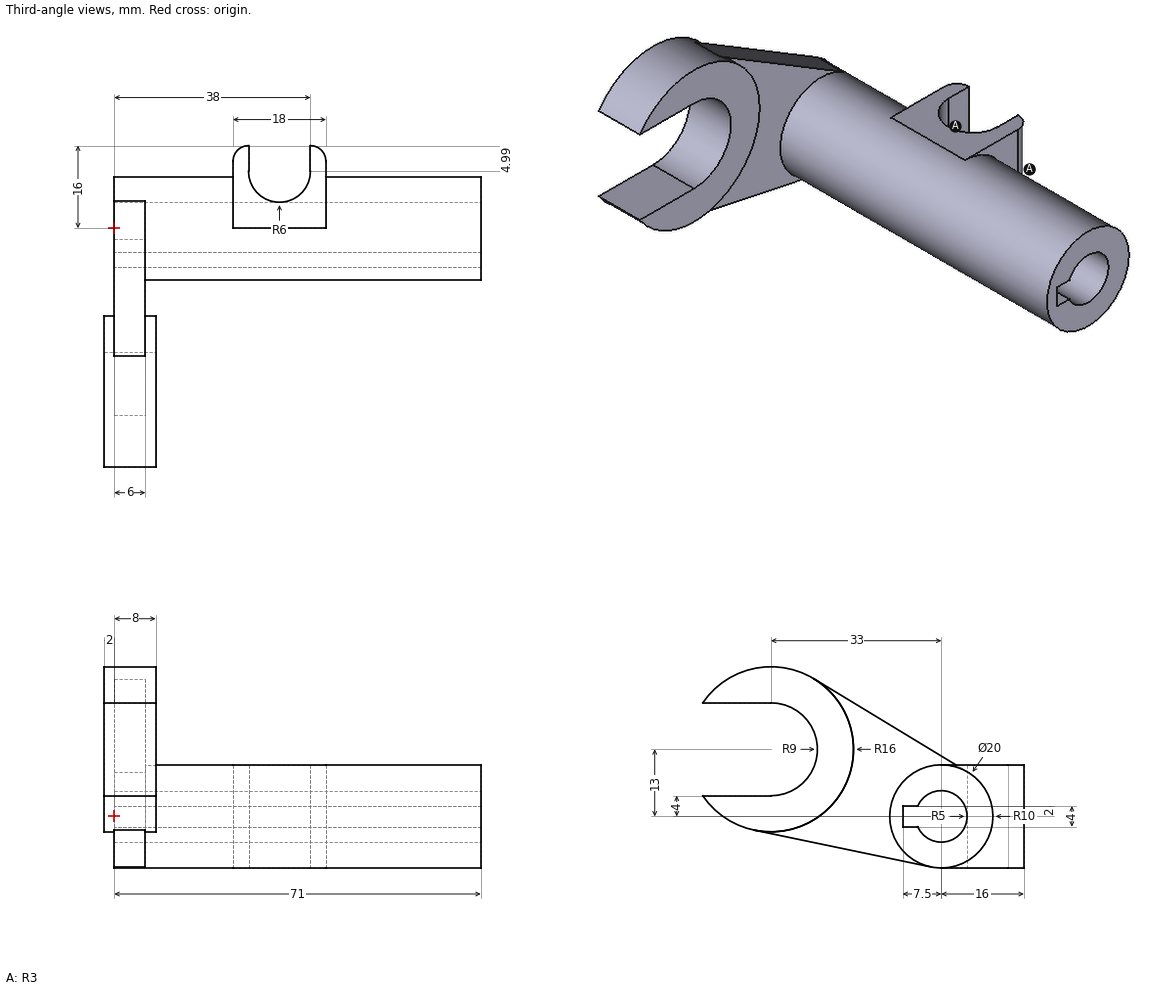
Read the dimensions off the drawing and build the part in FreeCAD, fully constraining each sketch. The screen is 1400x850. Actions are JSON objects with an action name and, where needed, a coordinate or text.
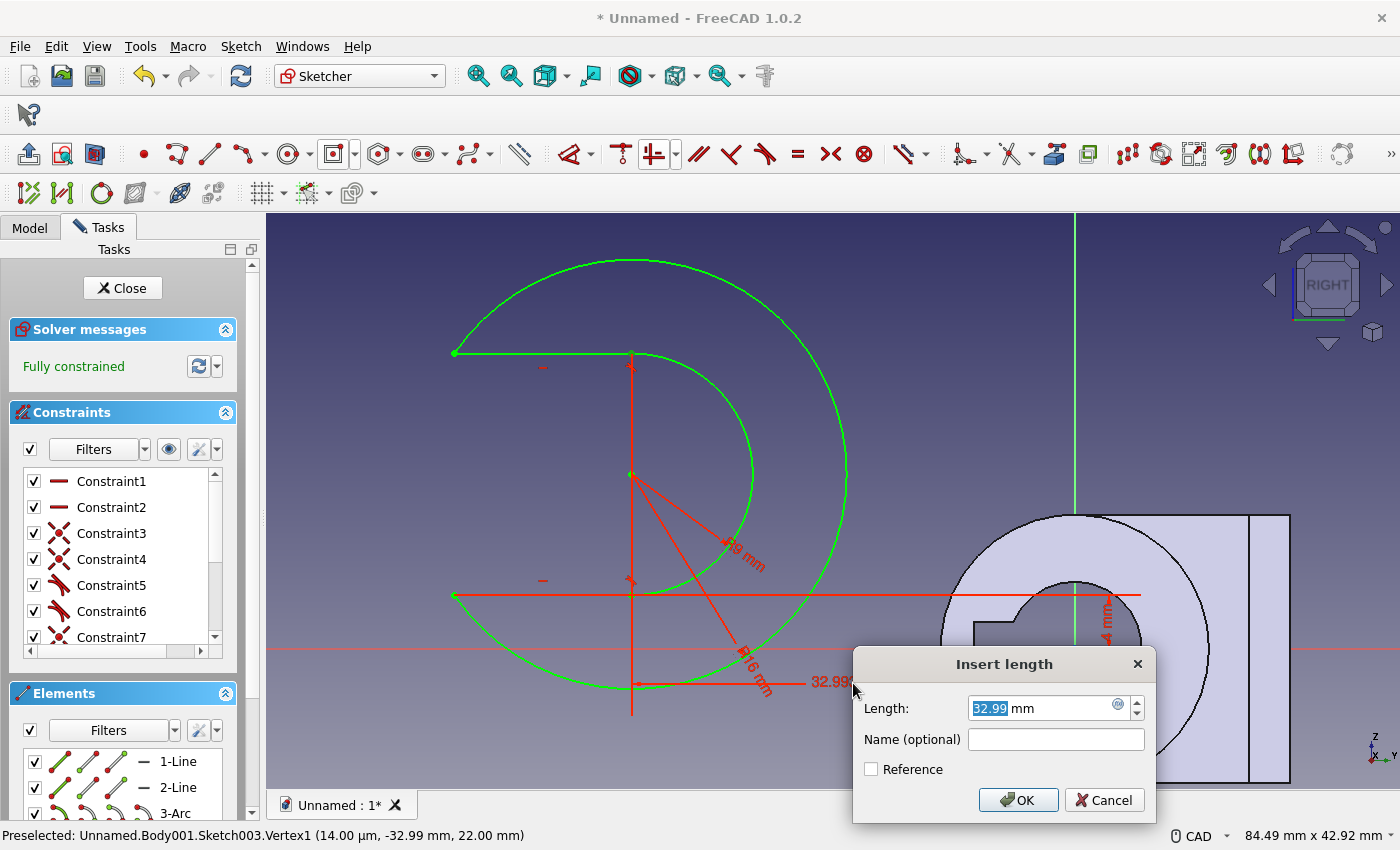
{"action": "type", "text": "33"}
{"action": "key", "text": "Return"}
{"action": "key", "text": "Escape"}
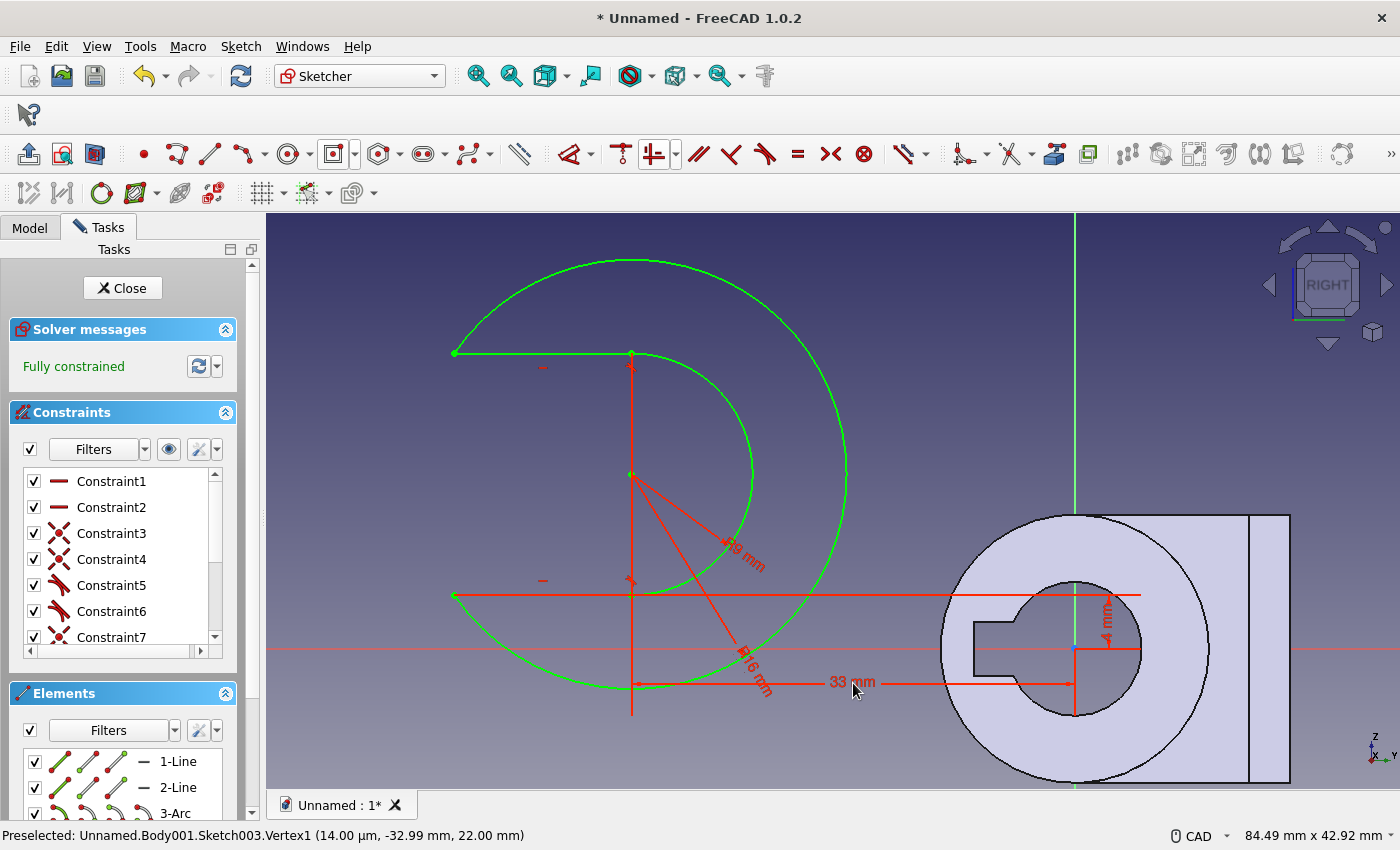
{"action": "left_click", "coordinate": [123, 288]}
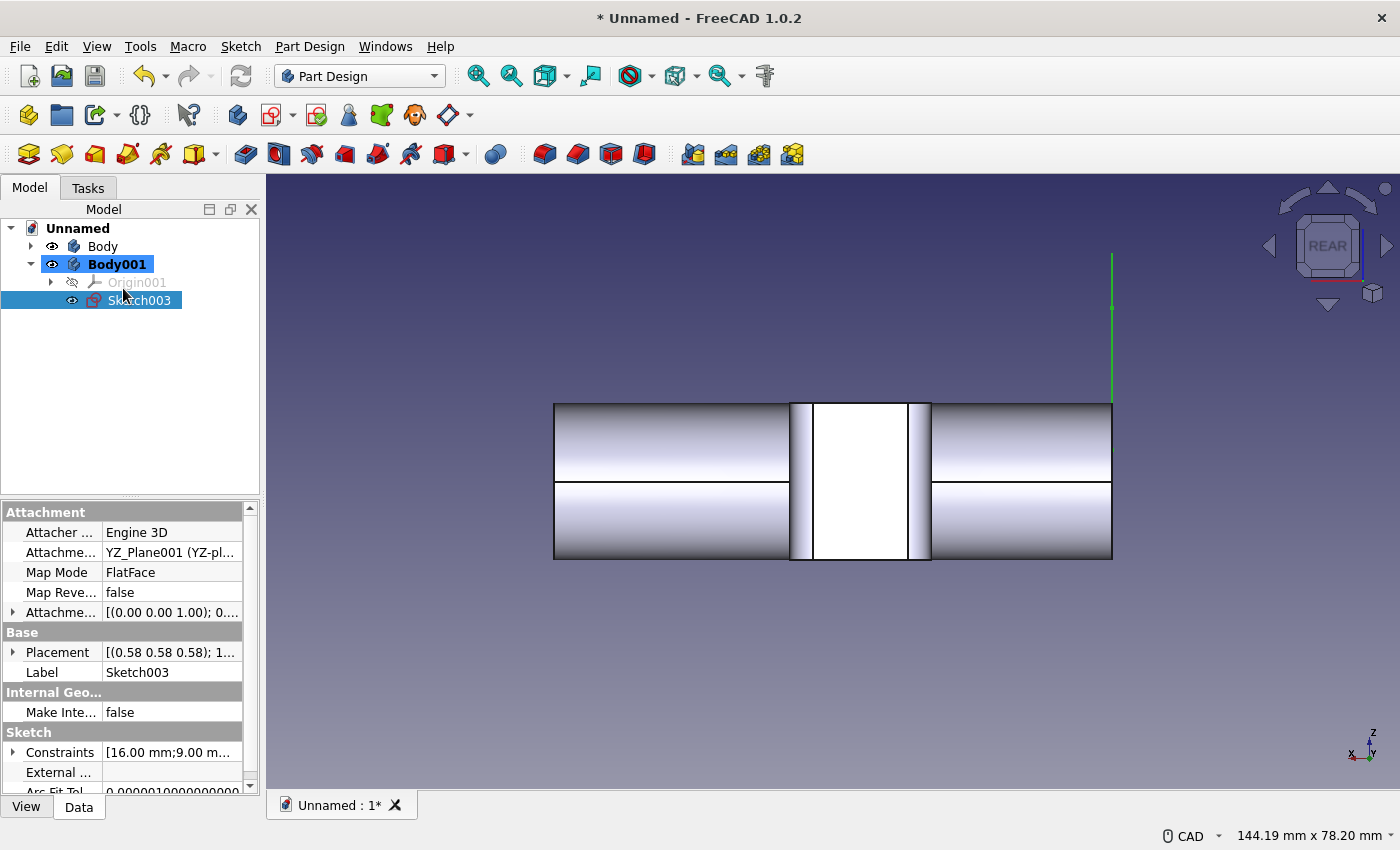
{"action": "left_click", "coordinate": [29, 154]}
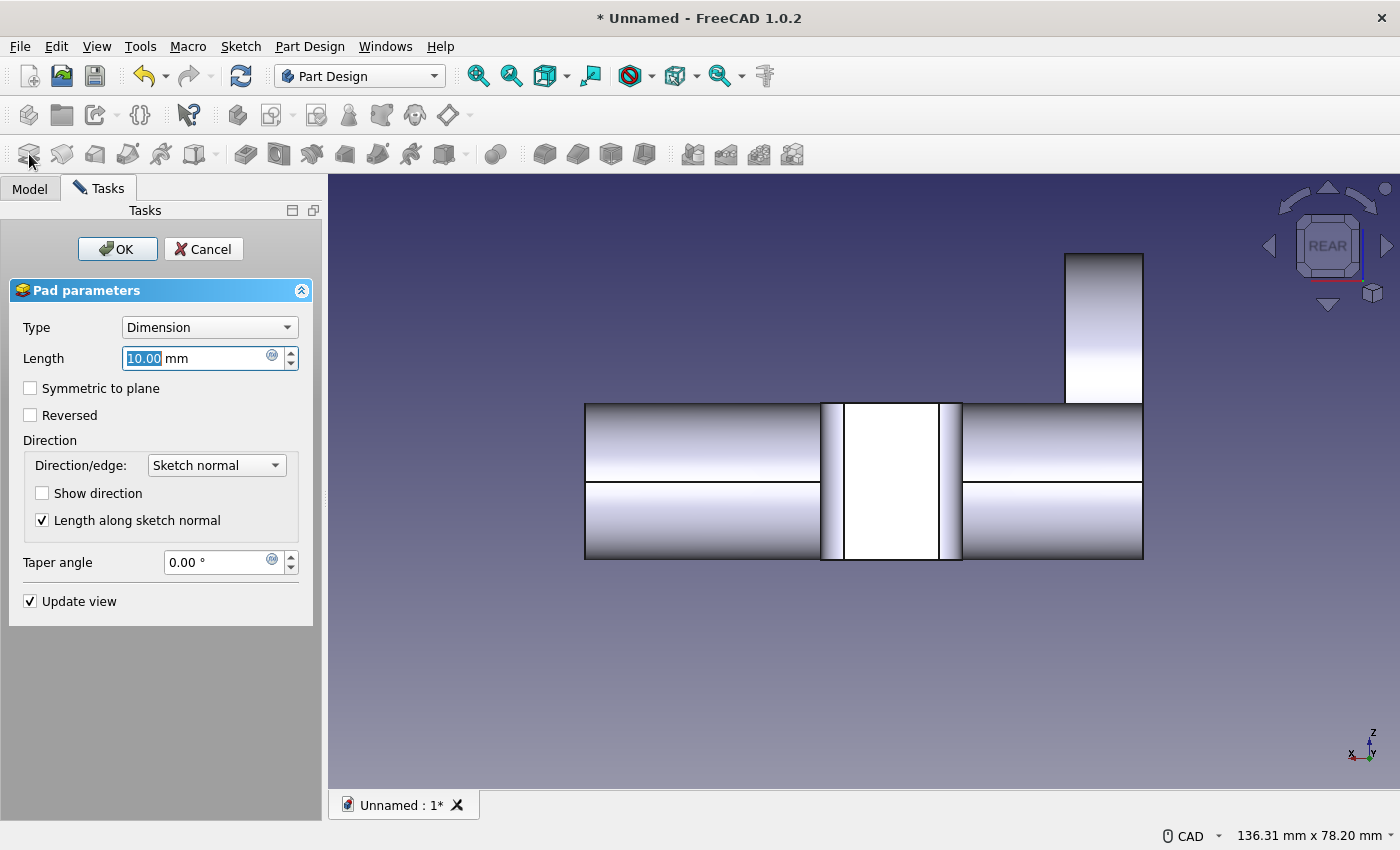
{"action": "left_click", "coordinate": [210, 328]}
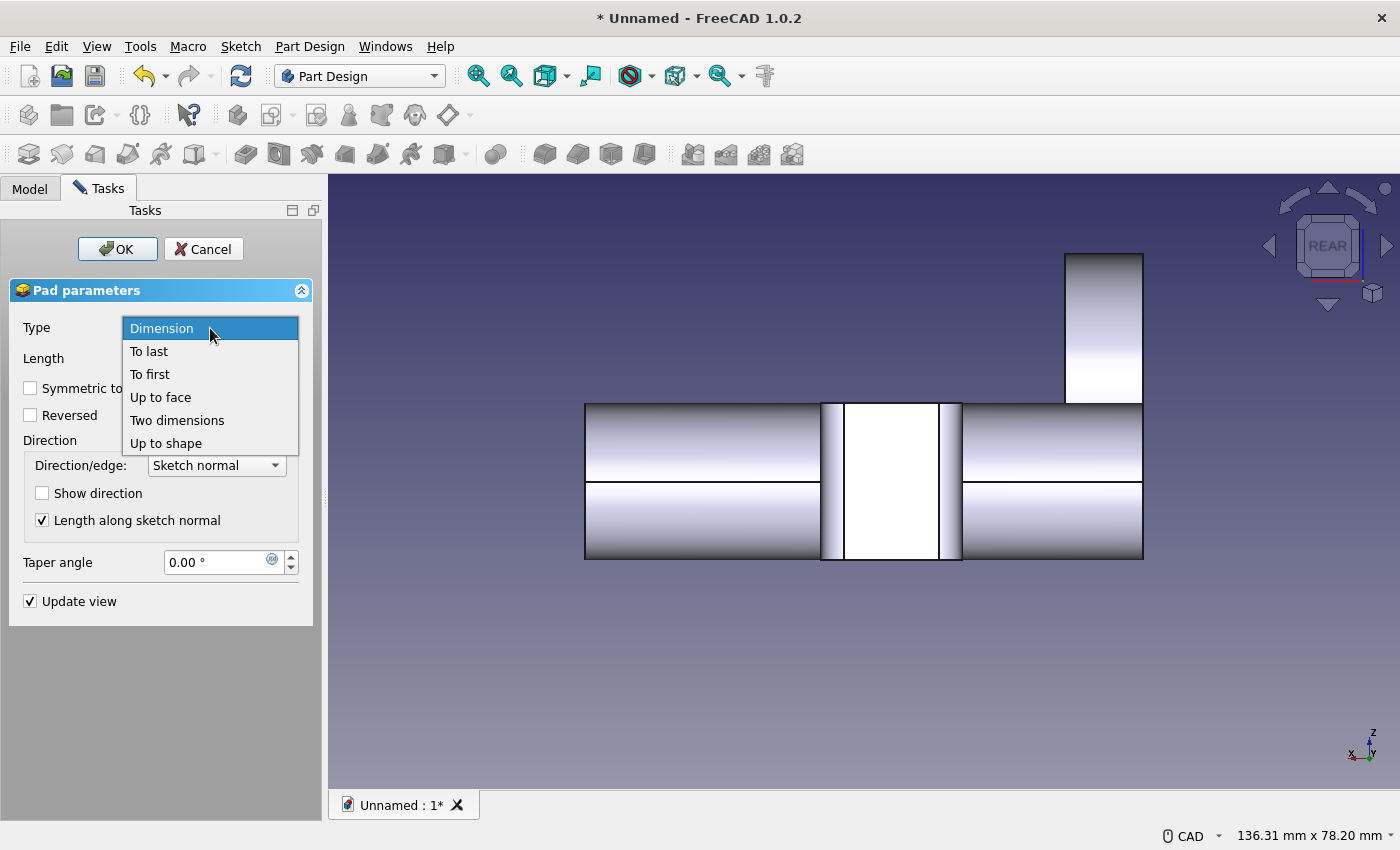
{"action": "left_click", "coordinate": [208, 420]}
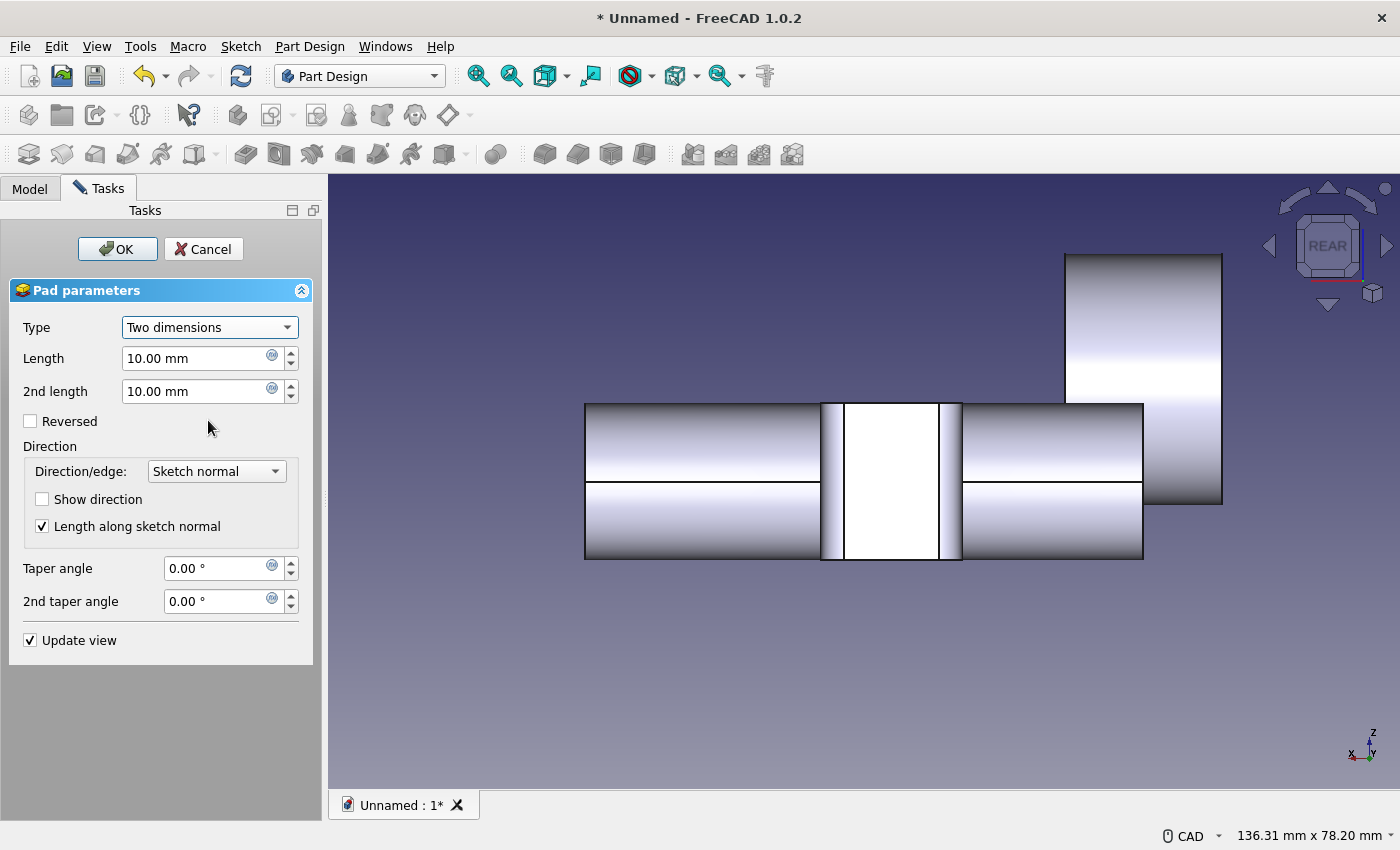
{"action": "triple_click", "coordinate": [204, 358]}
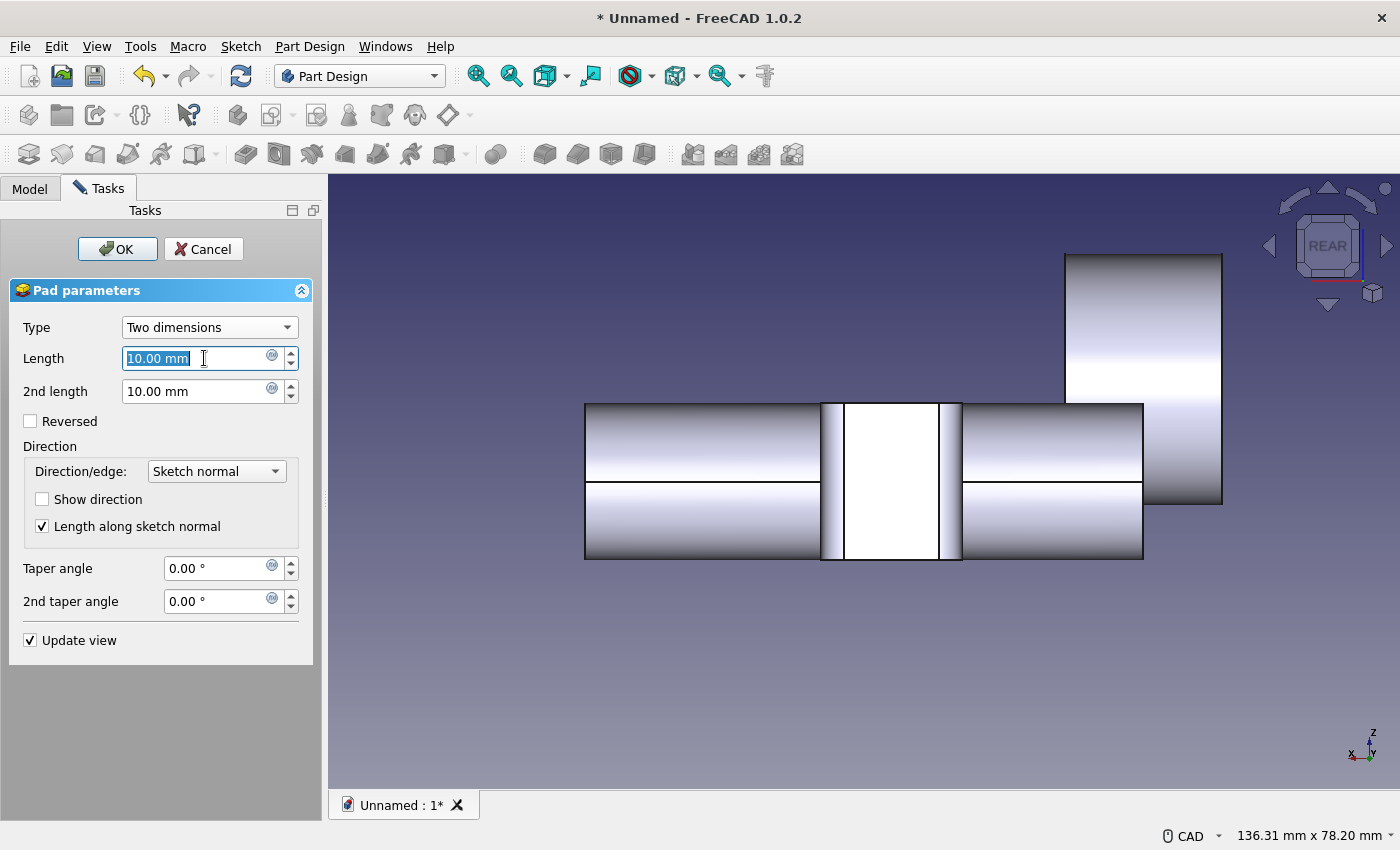
{"action": "type", "text": "2"}
{"action": "key", "text": "Tab"}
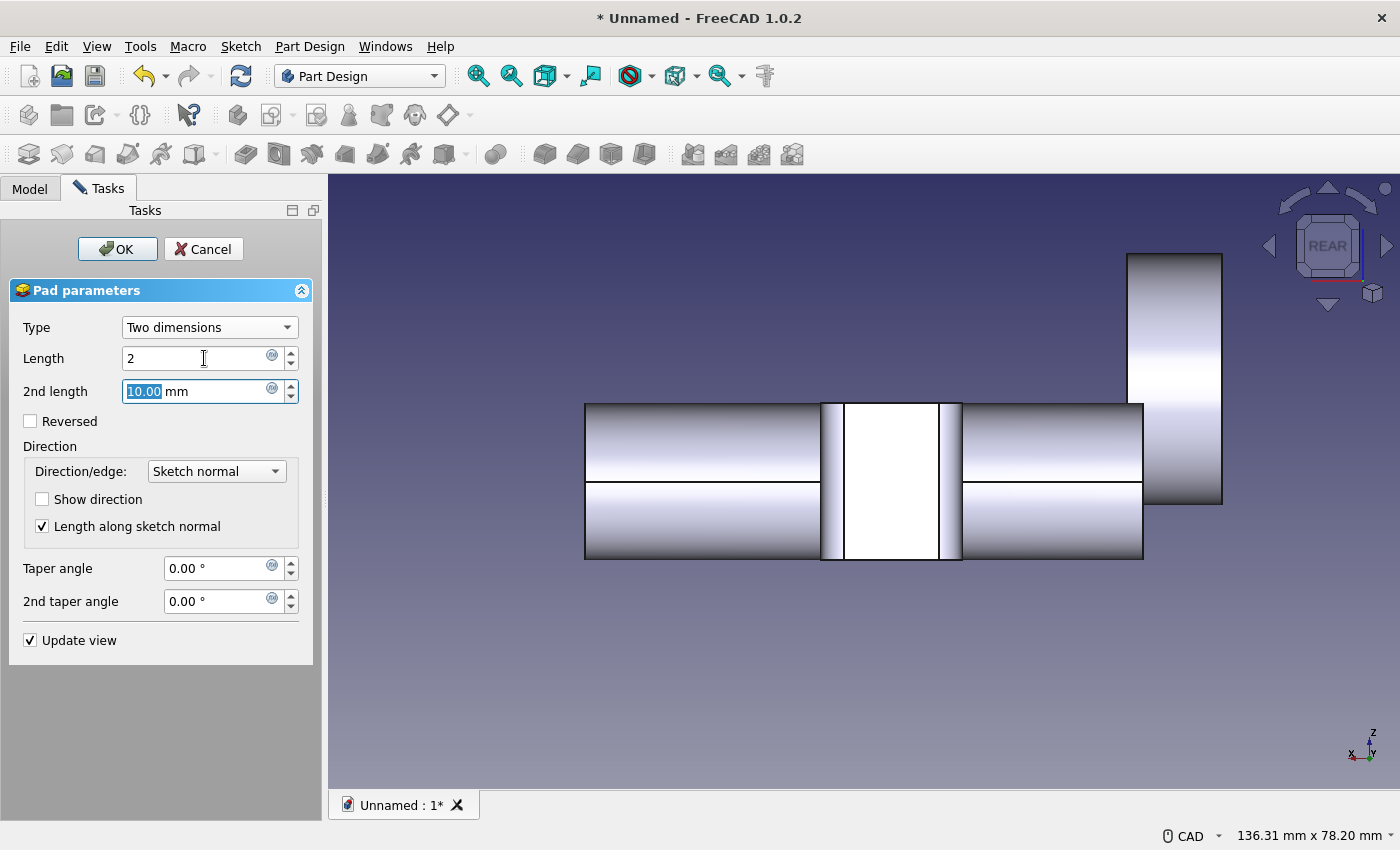
{"action": "type", "text": "8"}
{"action": "key", "text": "Tab"}